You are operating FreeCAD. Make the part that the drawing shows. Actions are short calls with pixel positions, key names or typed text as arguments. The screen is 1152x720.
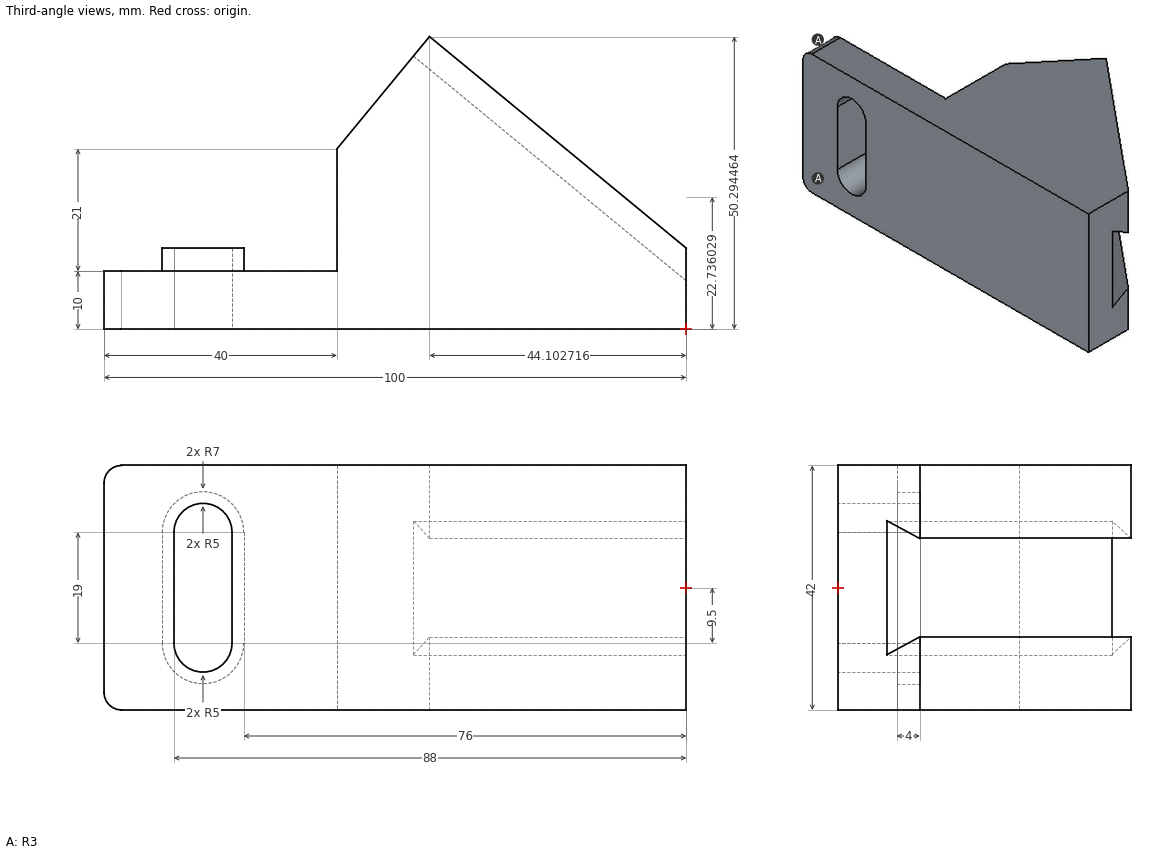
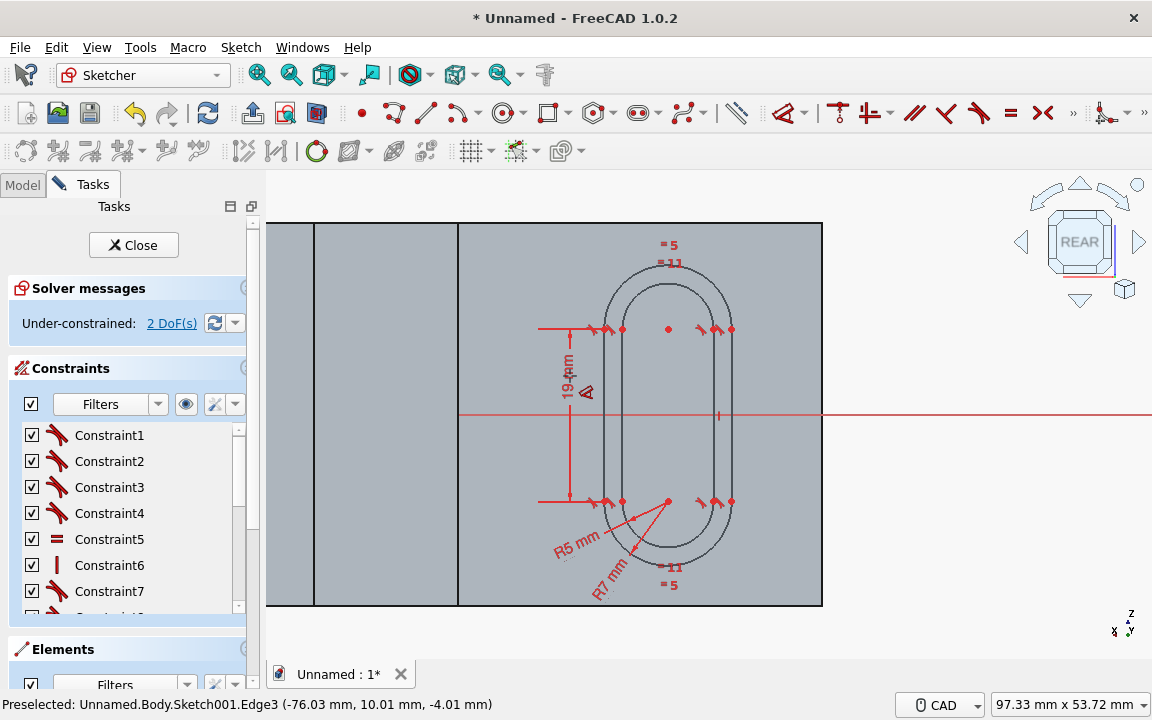
click(604, 502)
click(449, 536)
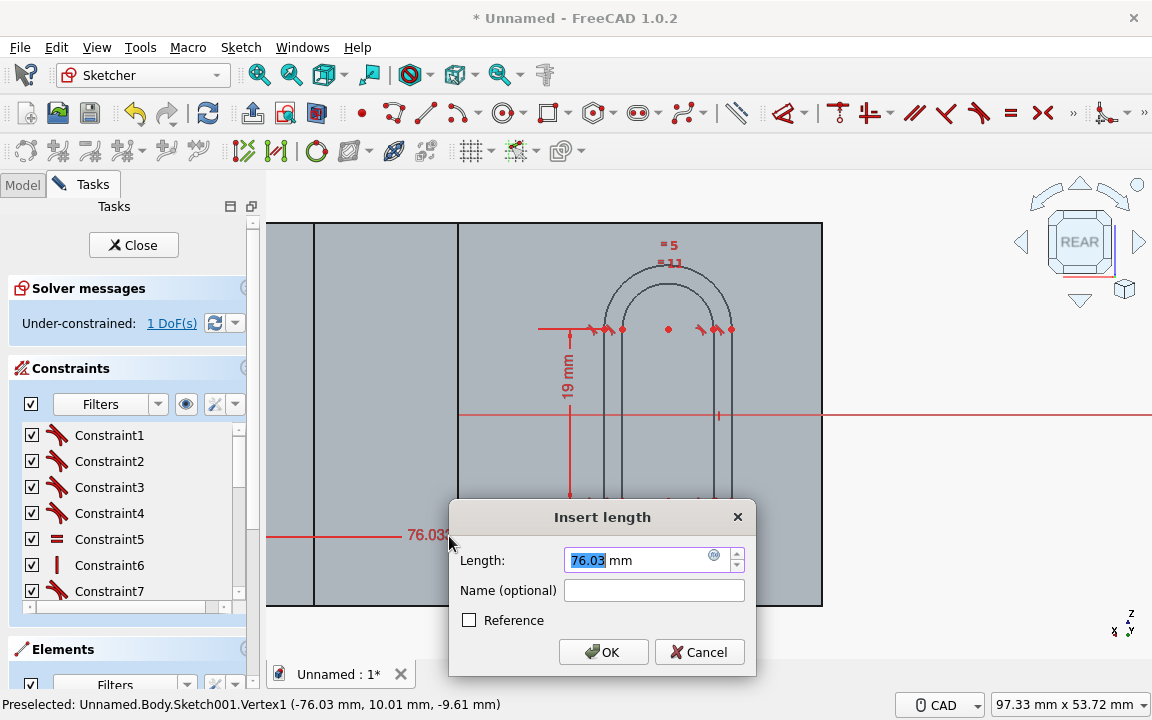
text(76)
key(Return)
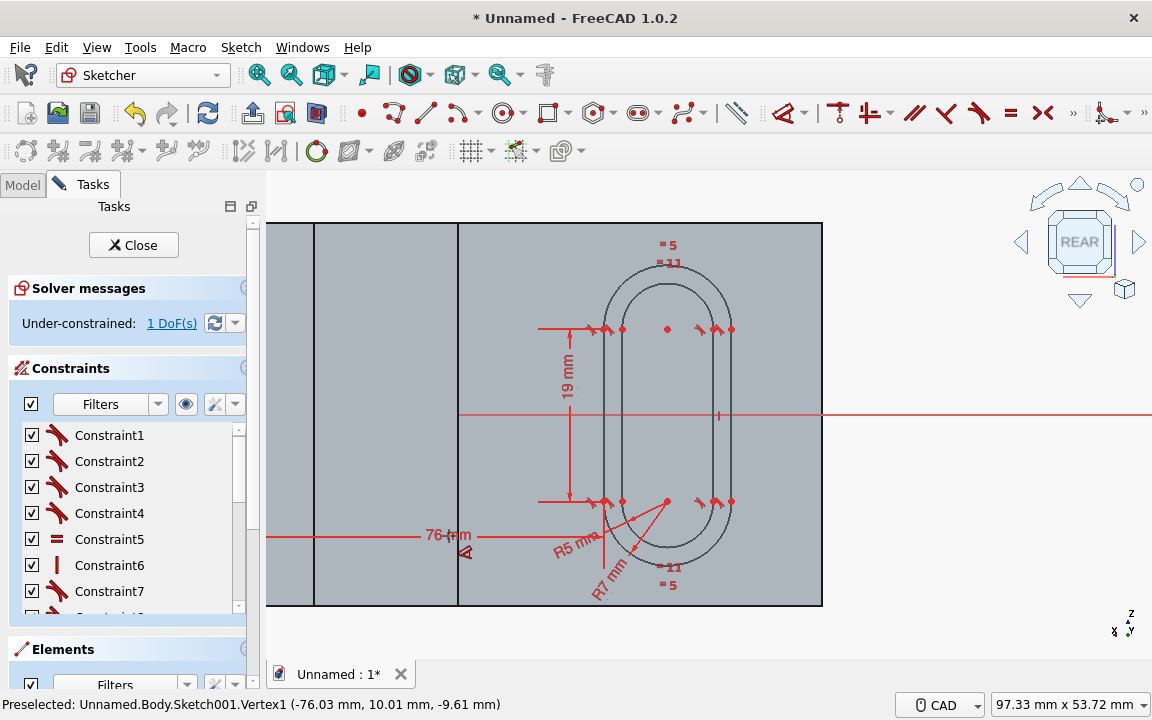
click(604, 502)
click(638, 458)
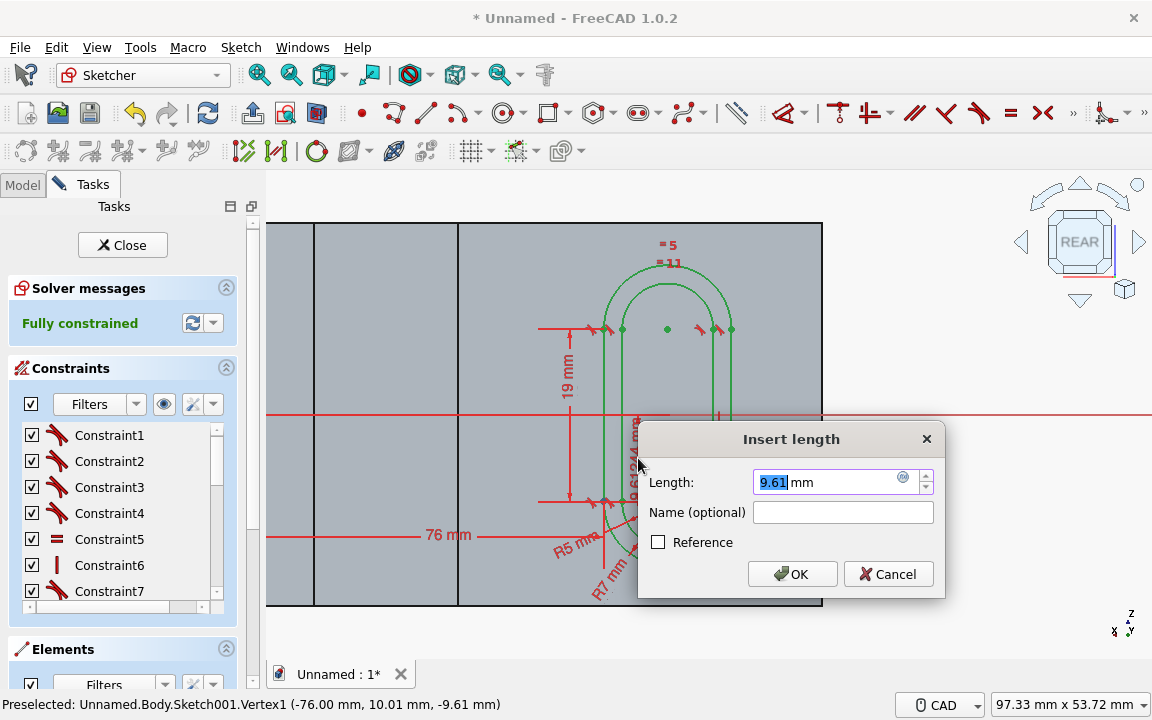
text(9.5)
key(Return)
key(Escape)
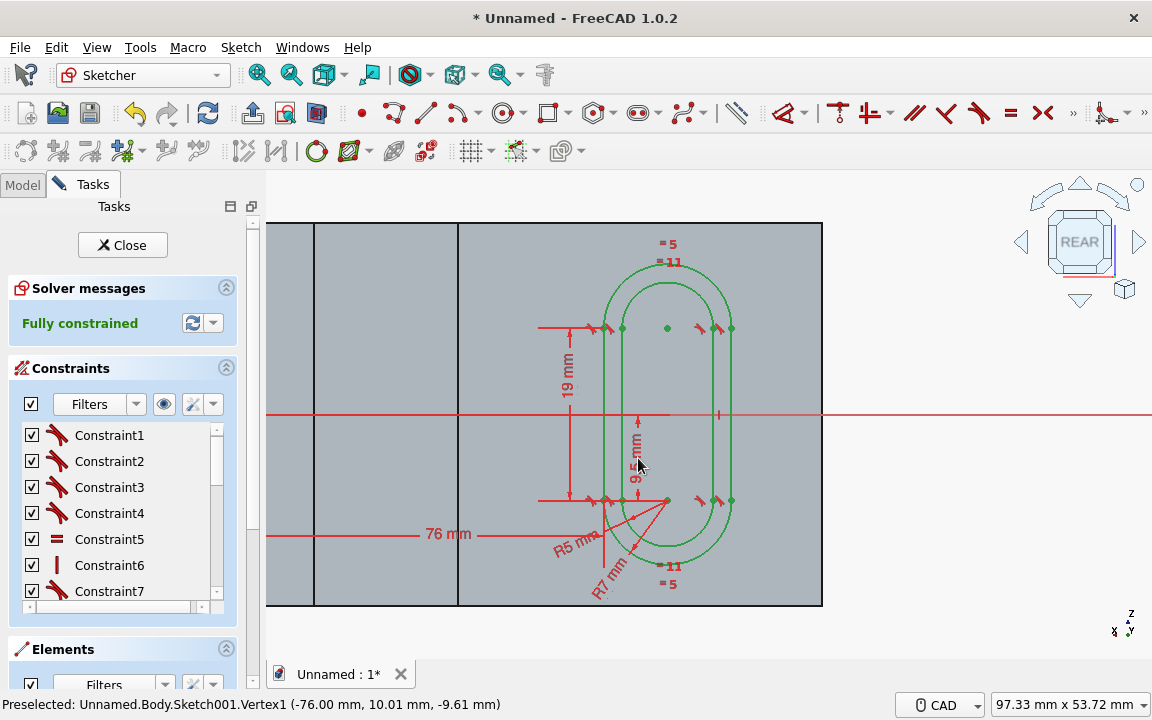
click(123, 245)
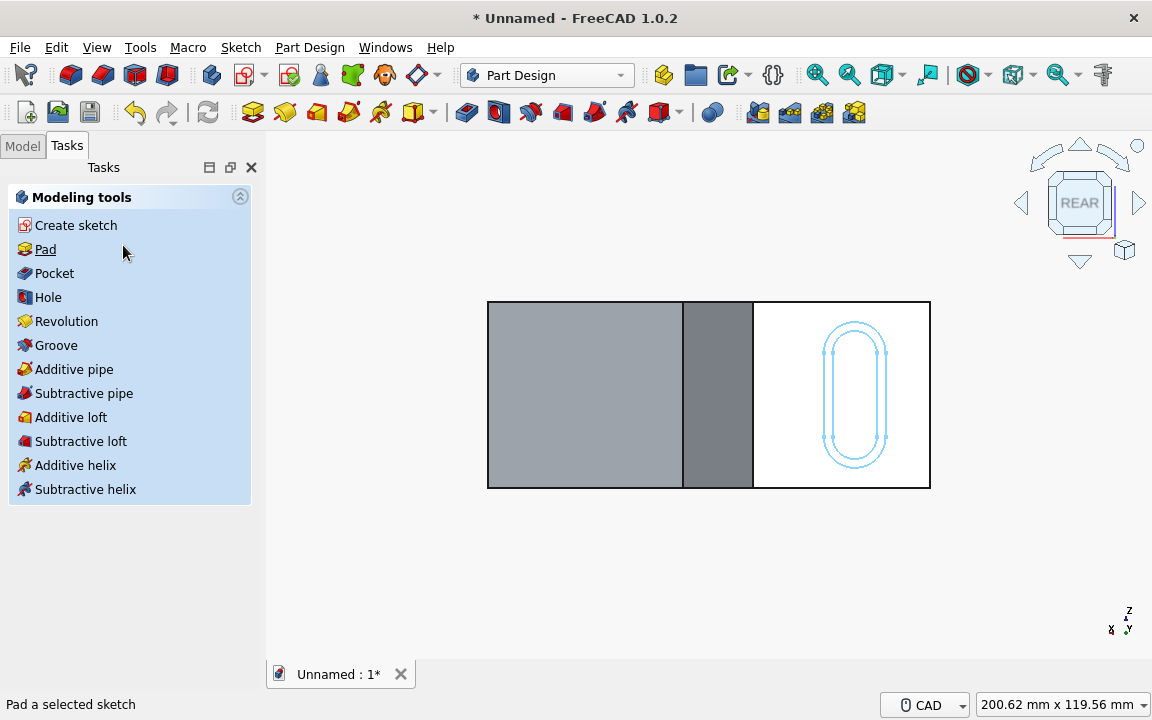
click(254, 112)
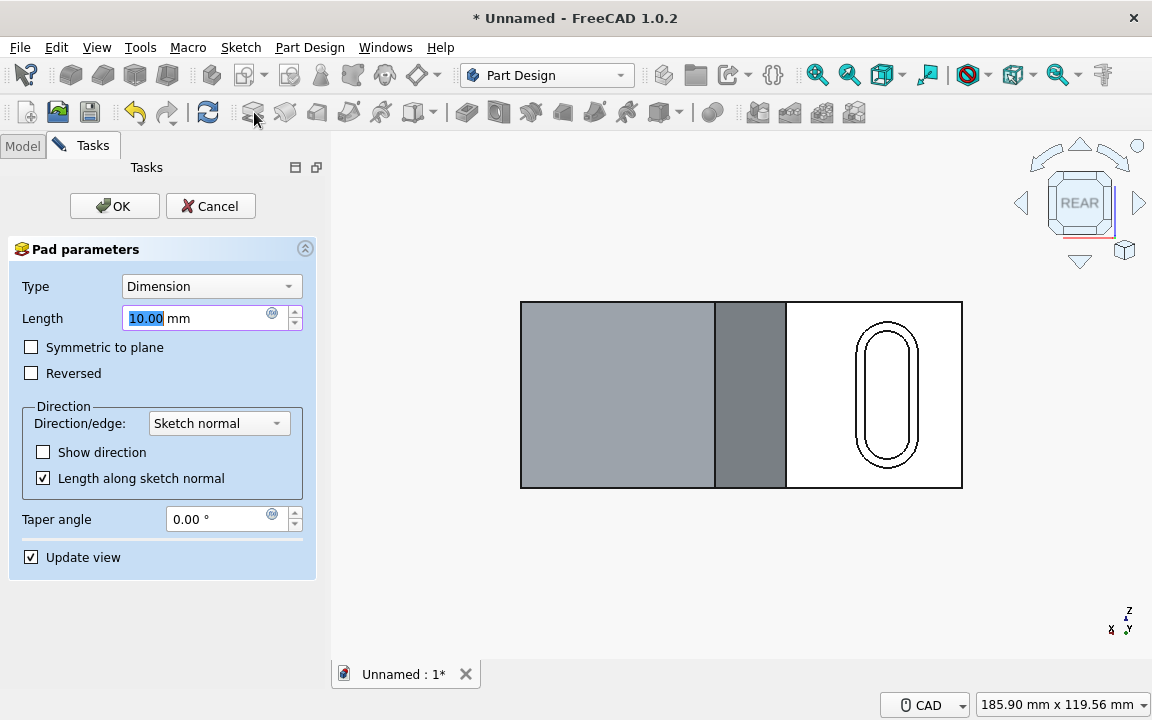
text(4)
key(Tab)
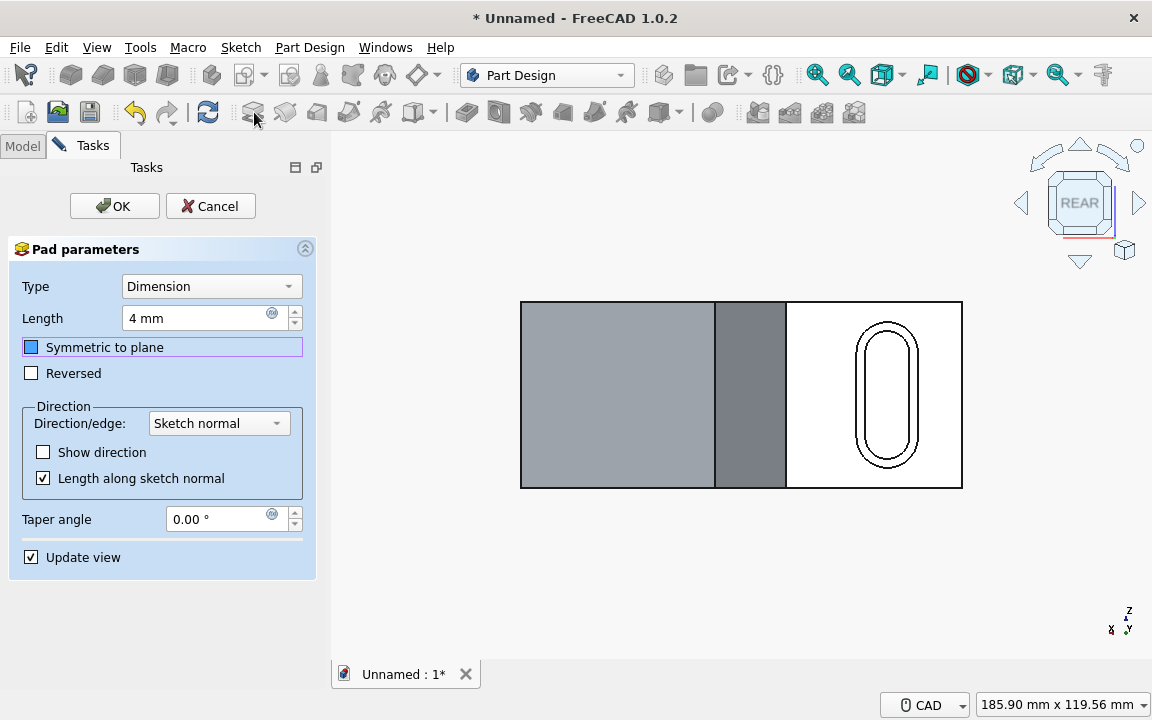
click(115, 206)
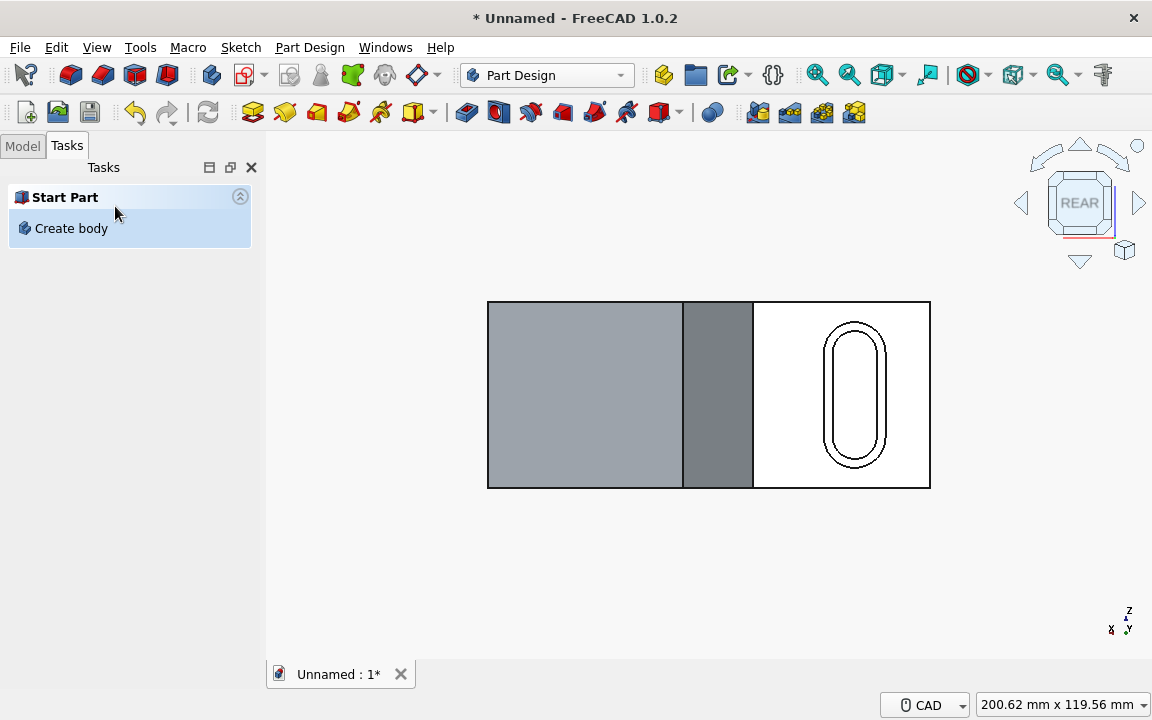
click(23, 145)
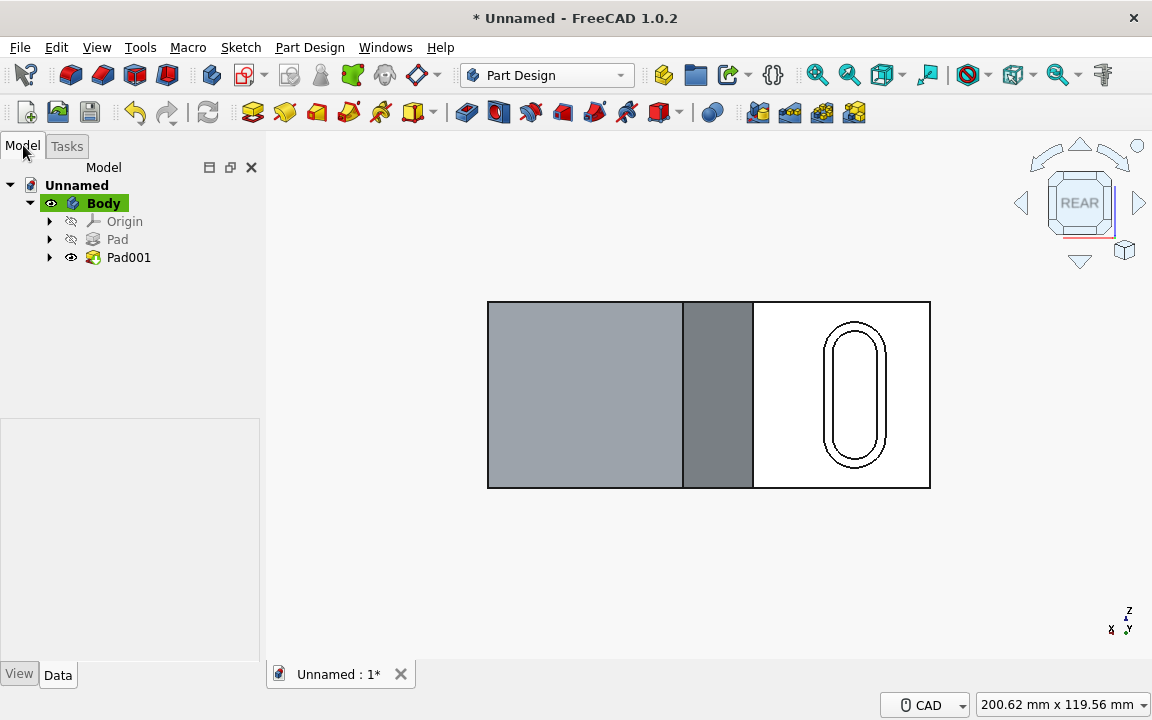
click(50, 221)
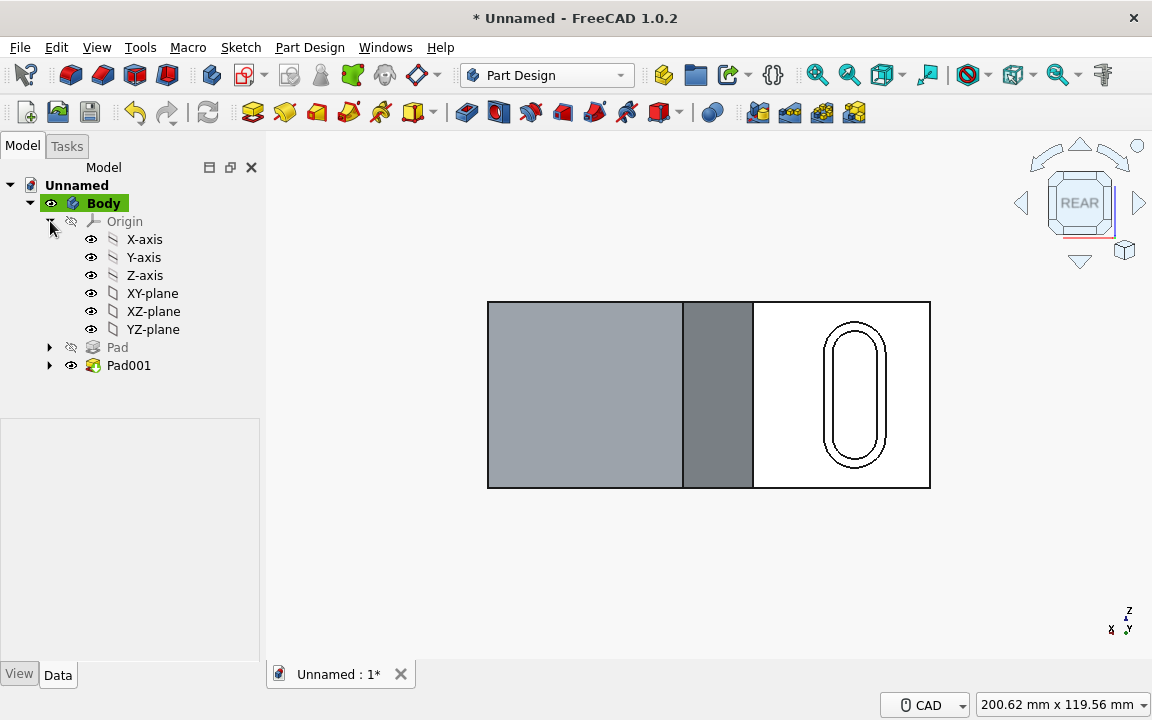
click(136, 311)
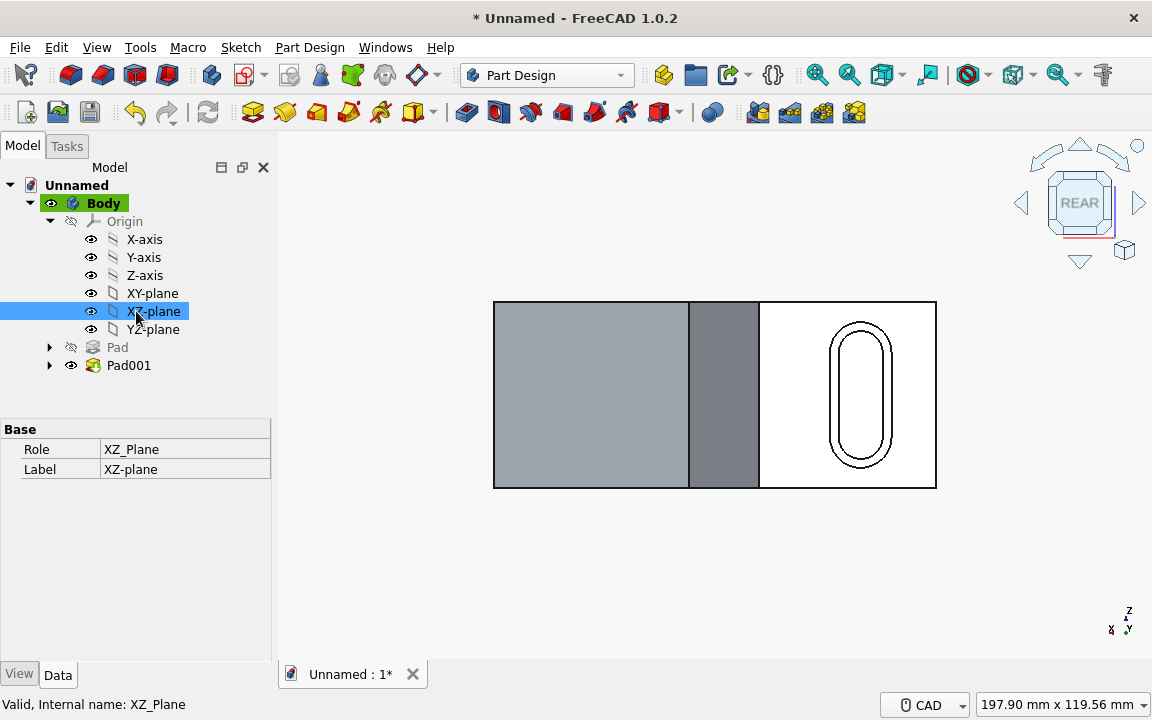
click(418, 76)